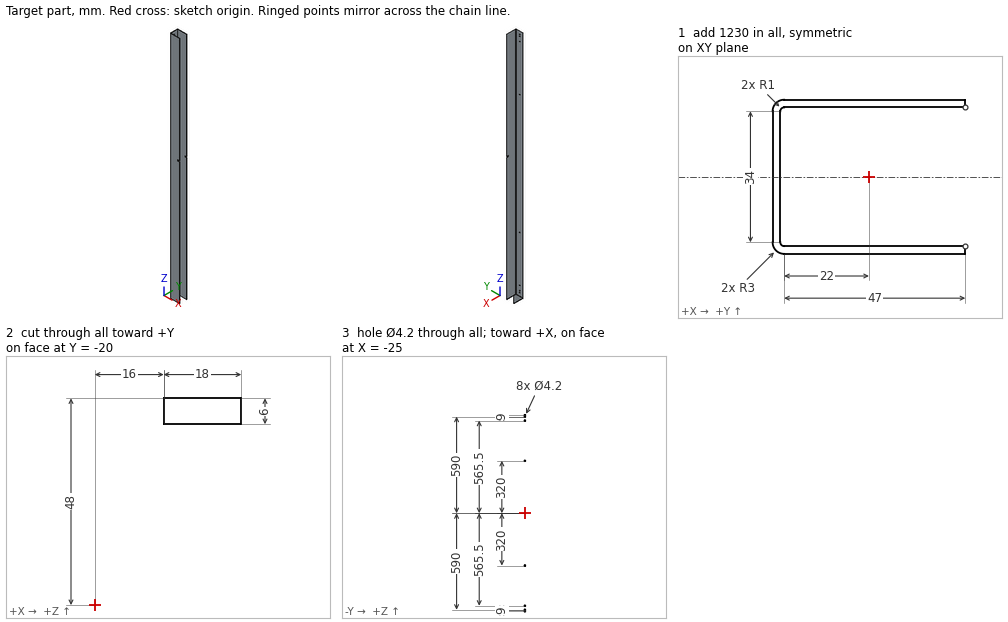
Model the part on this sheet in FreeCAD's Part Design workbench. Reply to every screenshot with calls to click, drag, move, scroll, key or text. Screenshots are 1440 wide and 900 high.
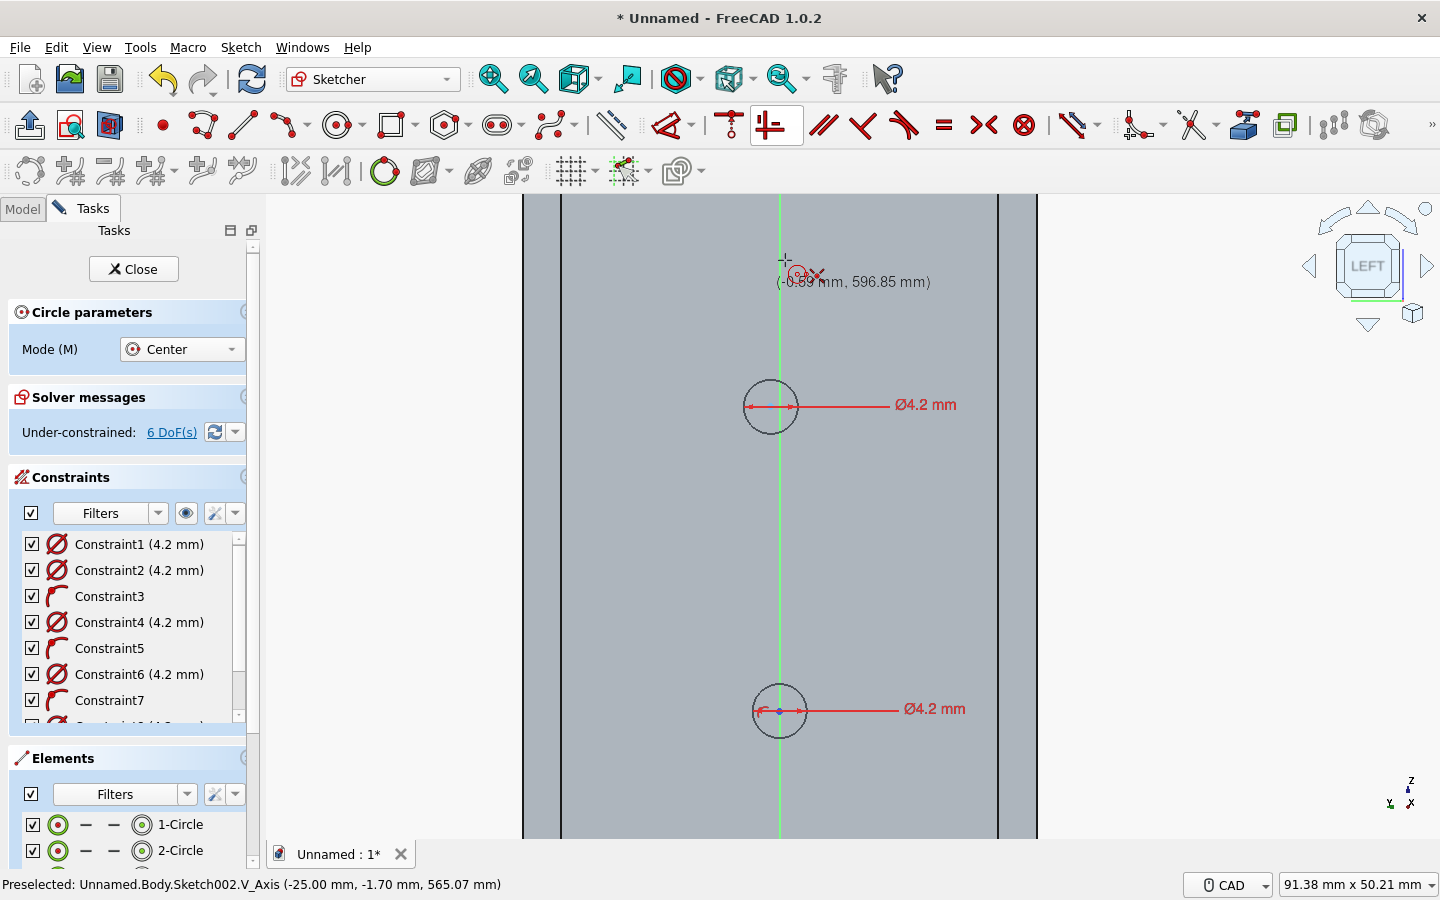
scroll(785, 260, down, 17)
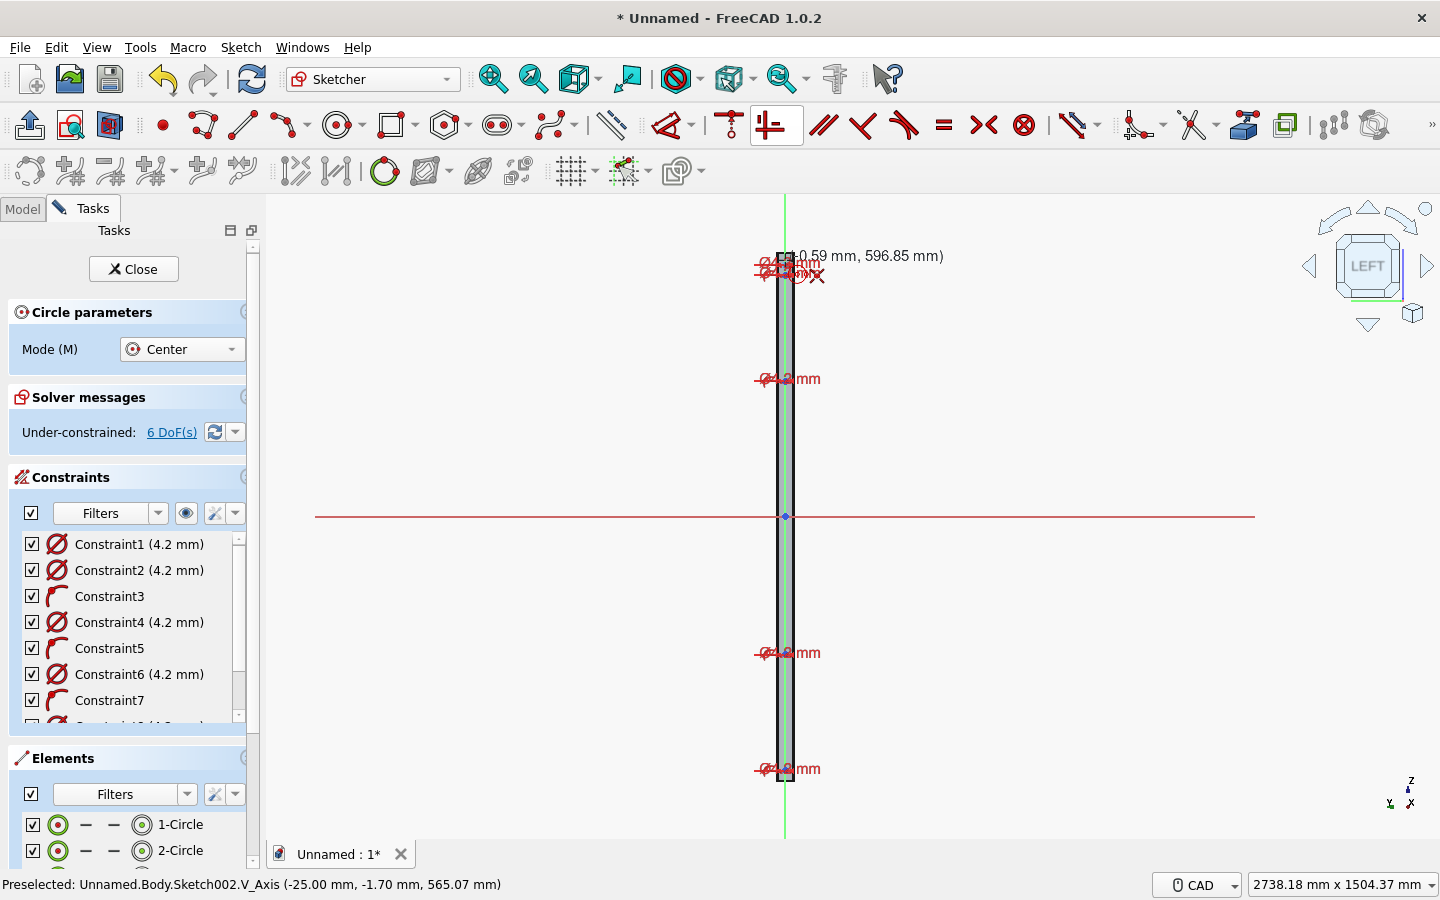
scroll(785, 260, up, 9)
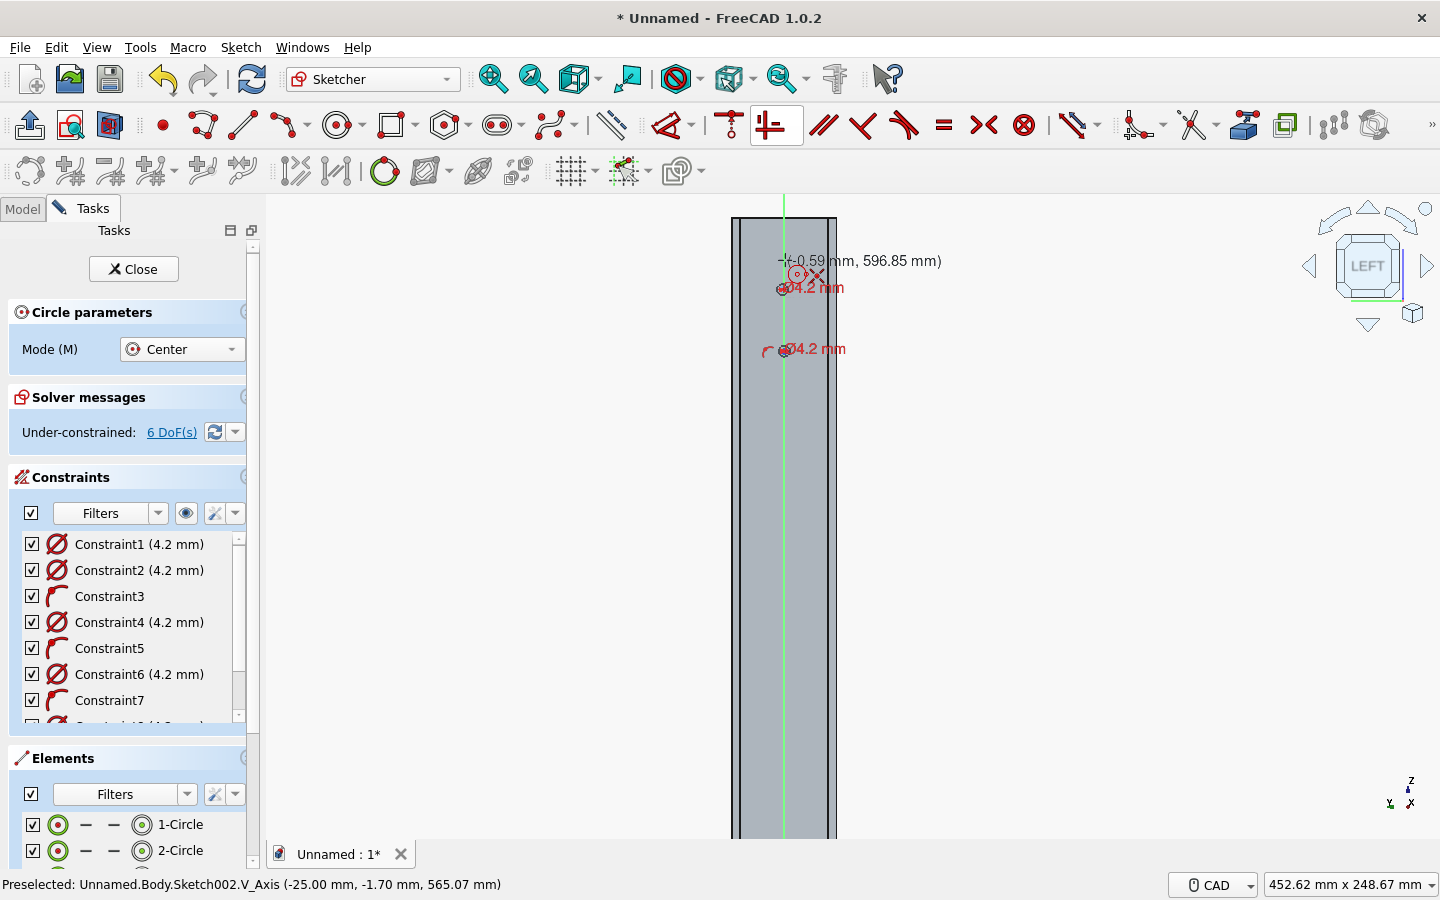
click(784, 260)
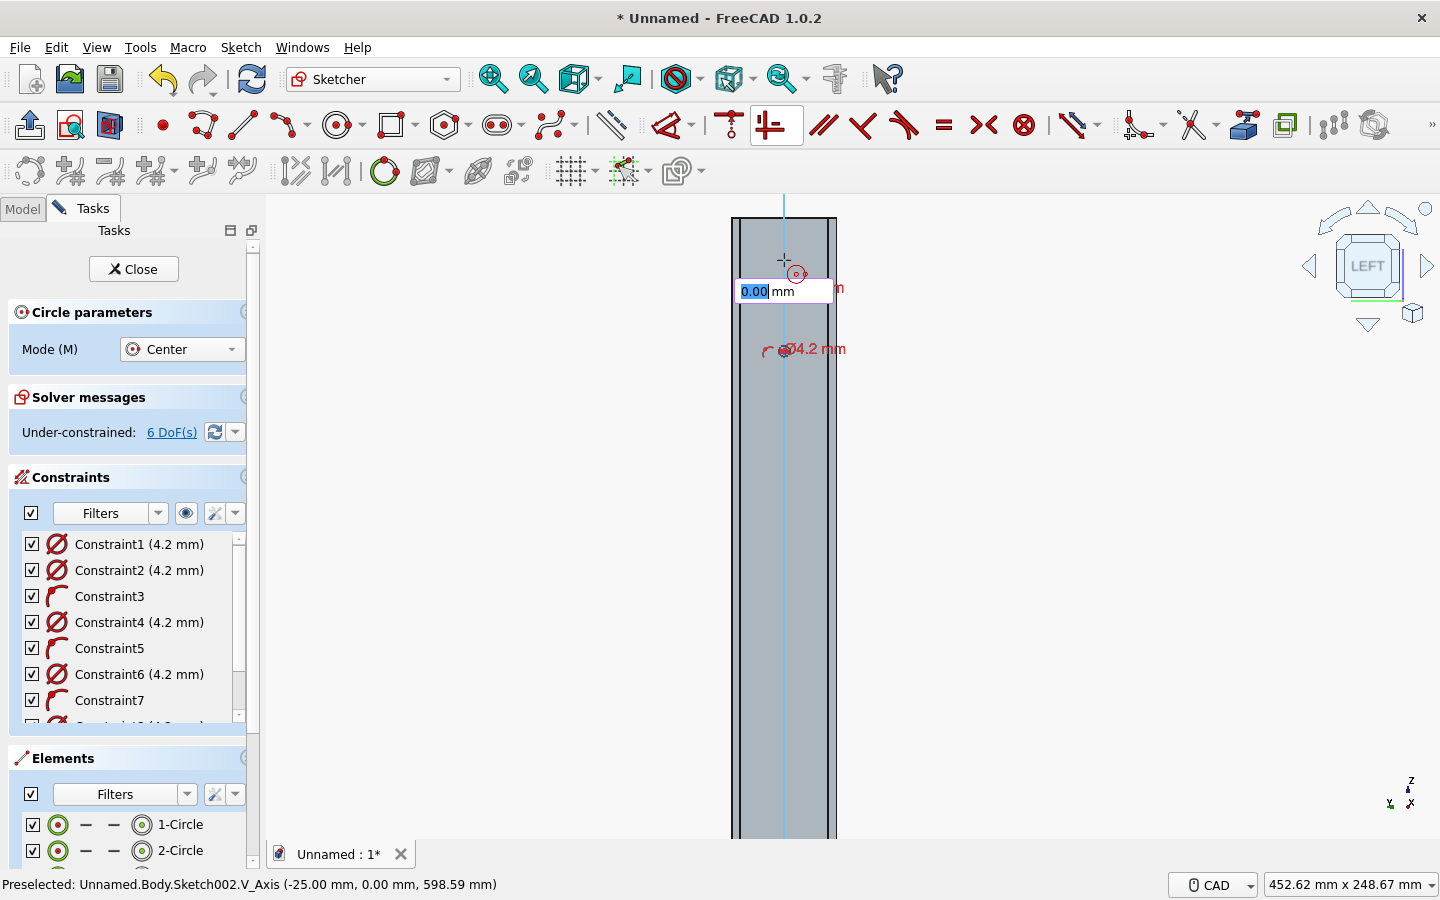
scroll(789, 258, up, 6)
move(789, 258)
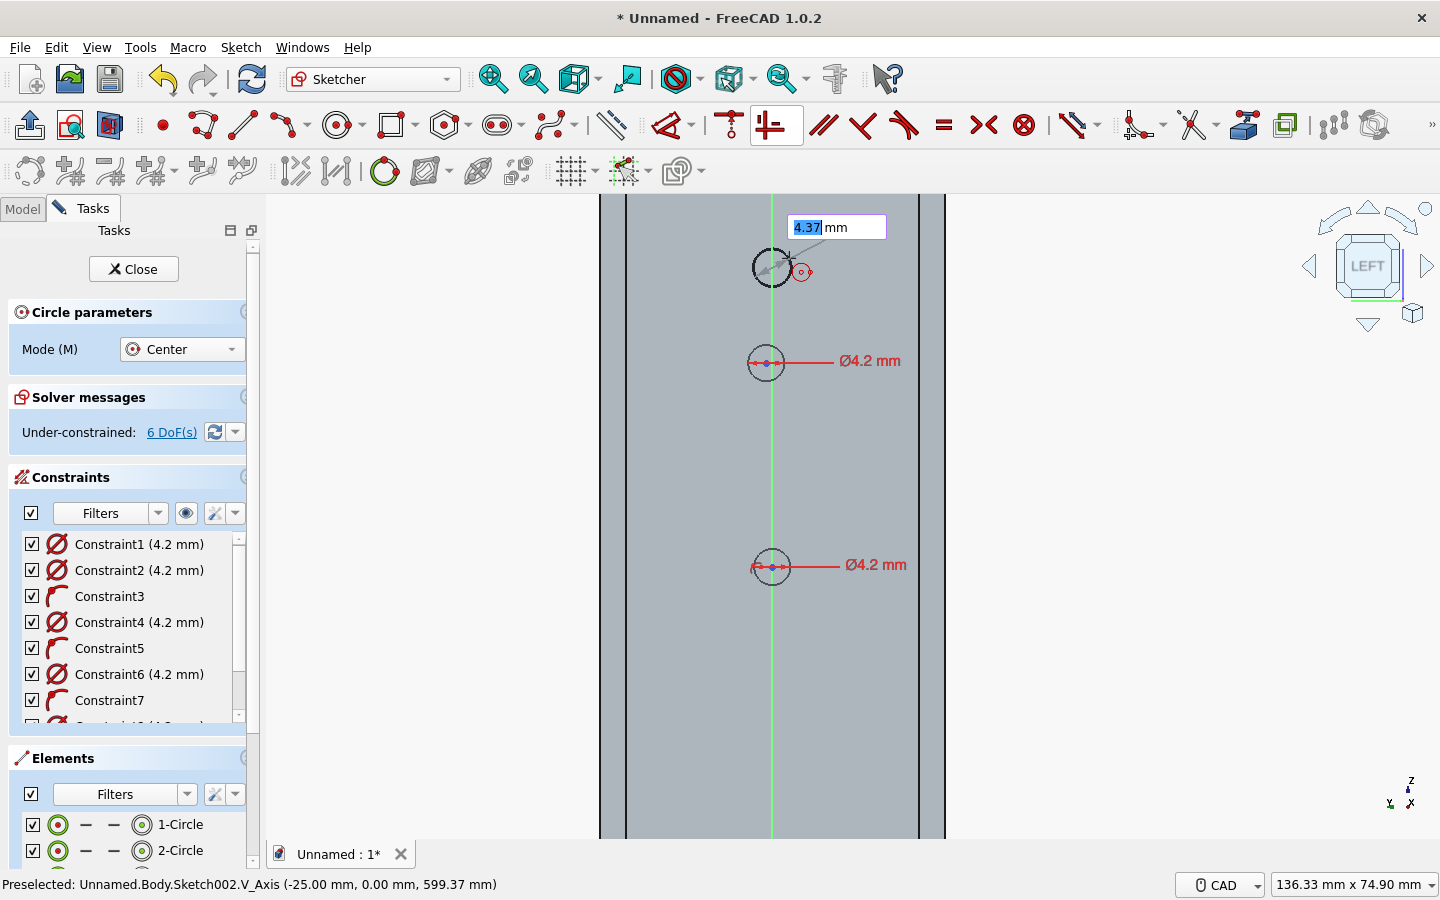
text(4.2)
key(Return)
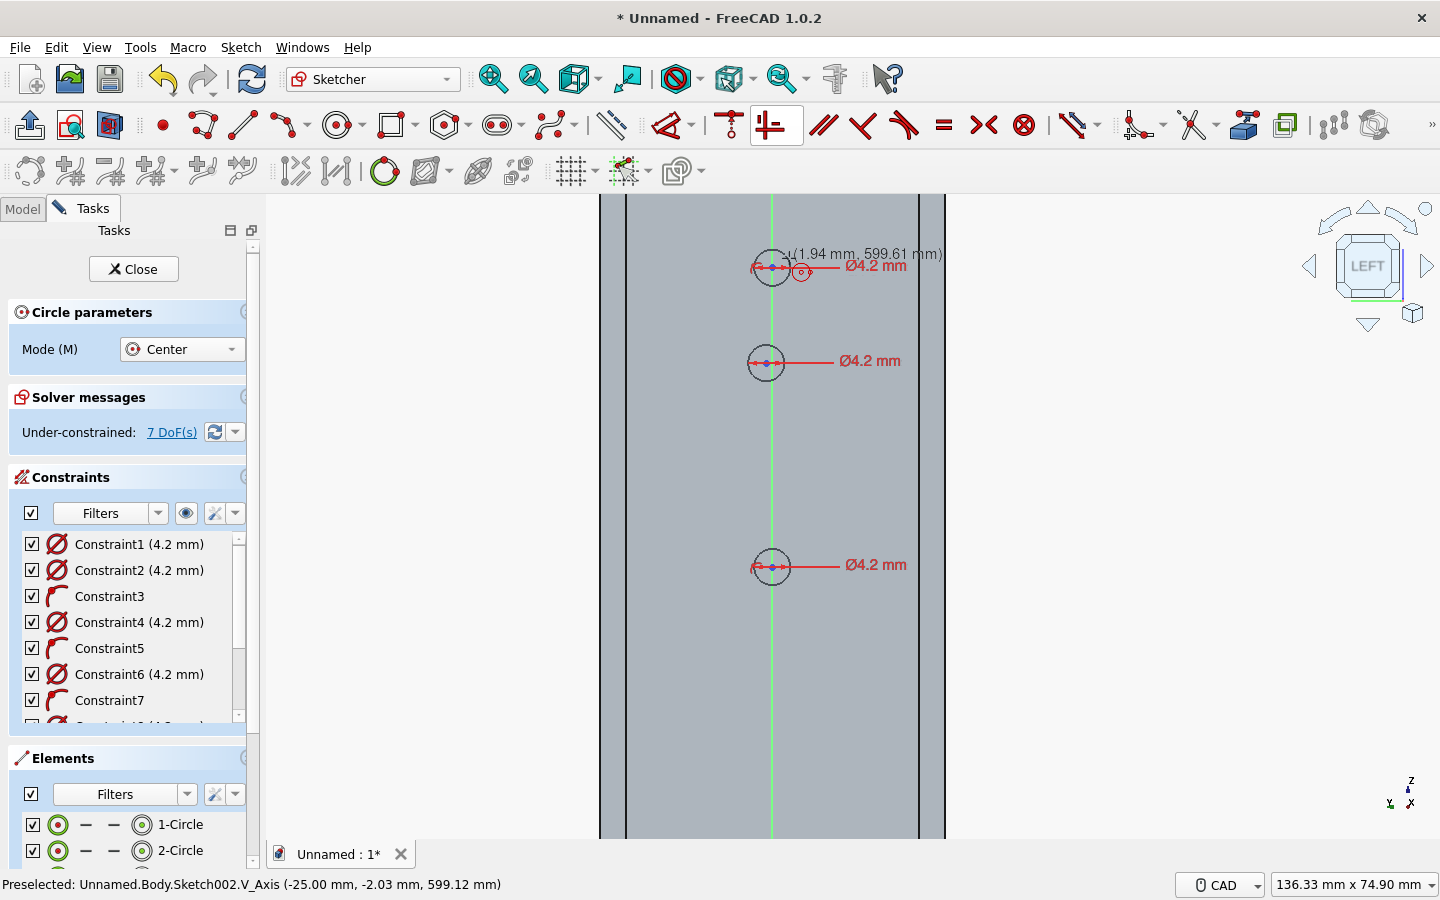
scroll(785, 259, down, 15)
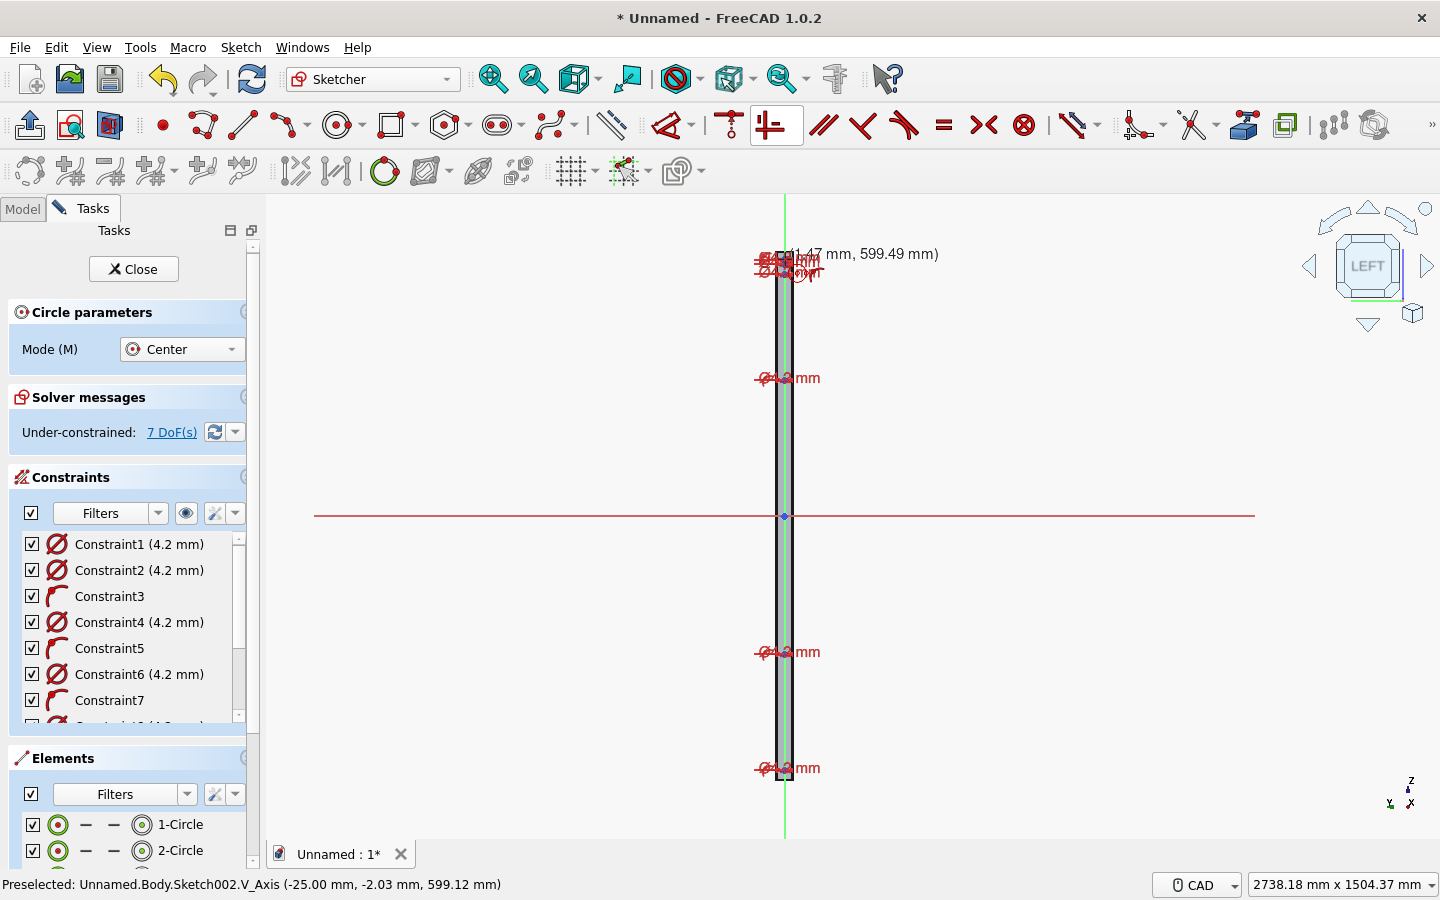
scroll(785, 773, up, 17)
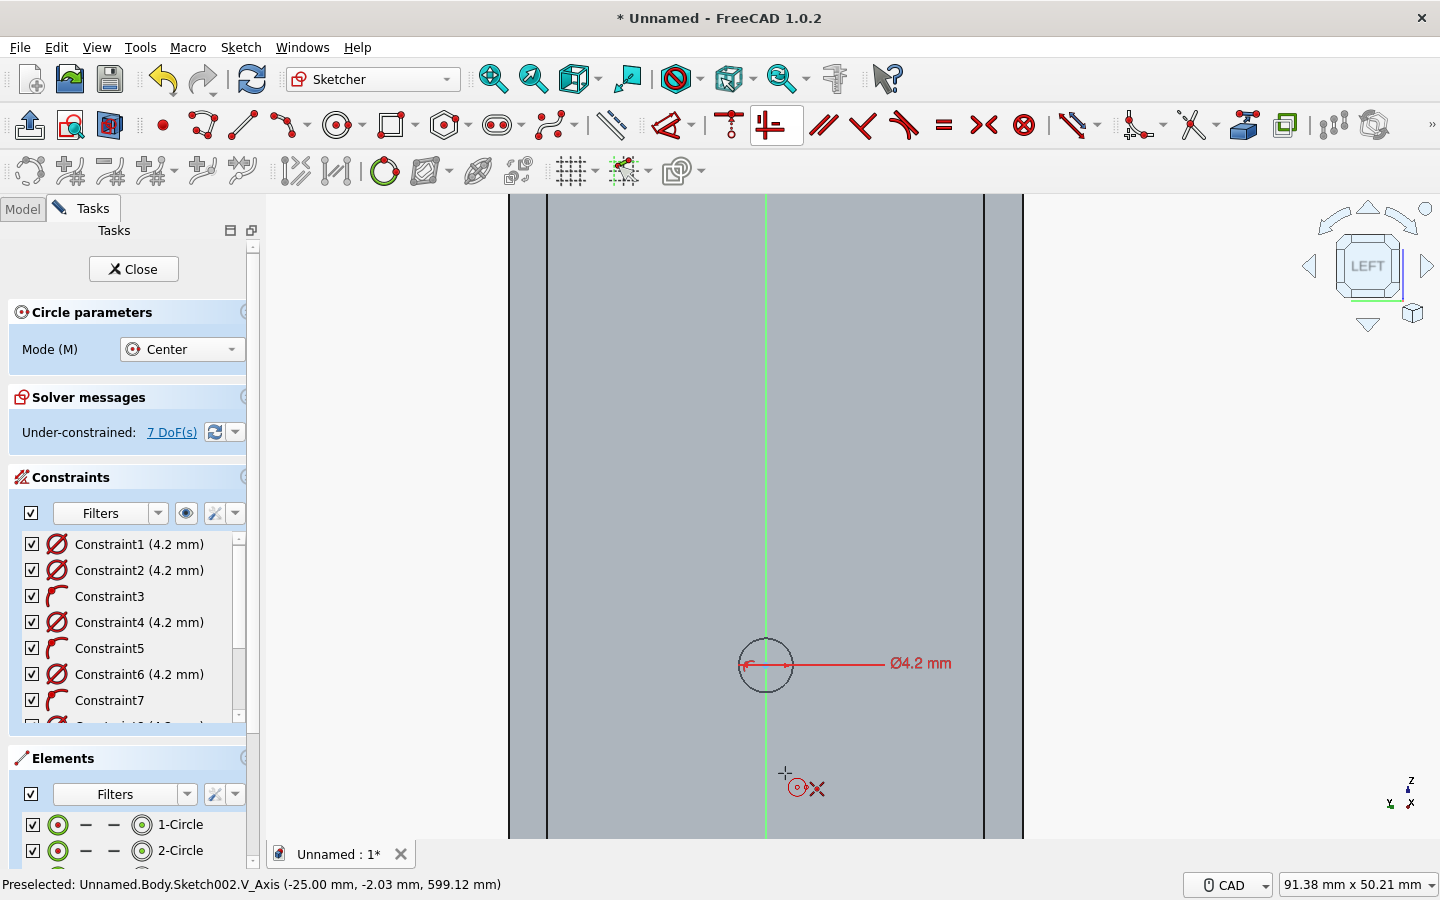
scroll(785, 774, down, 17)